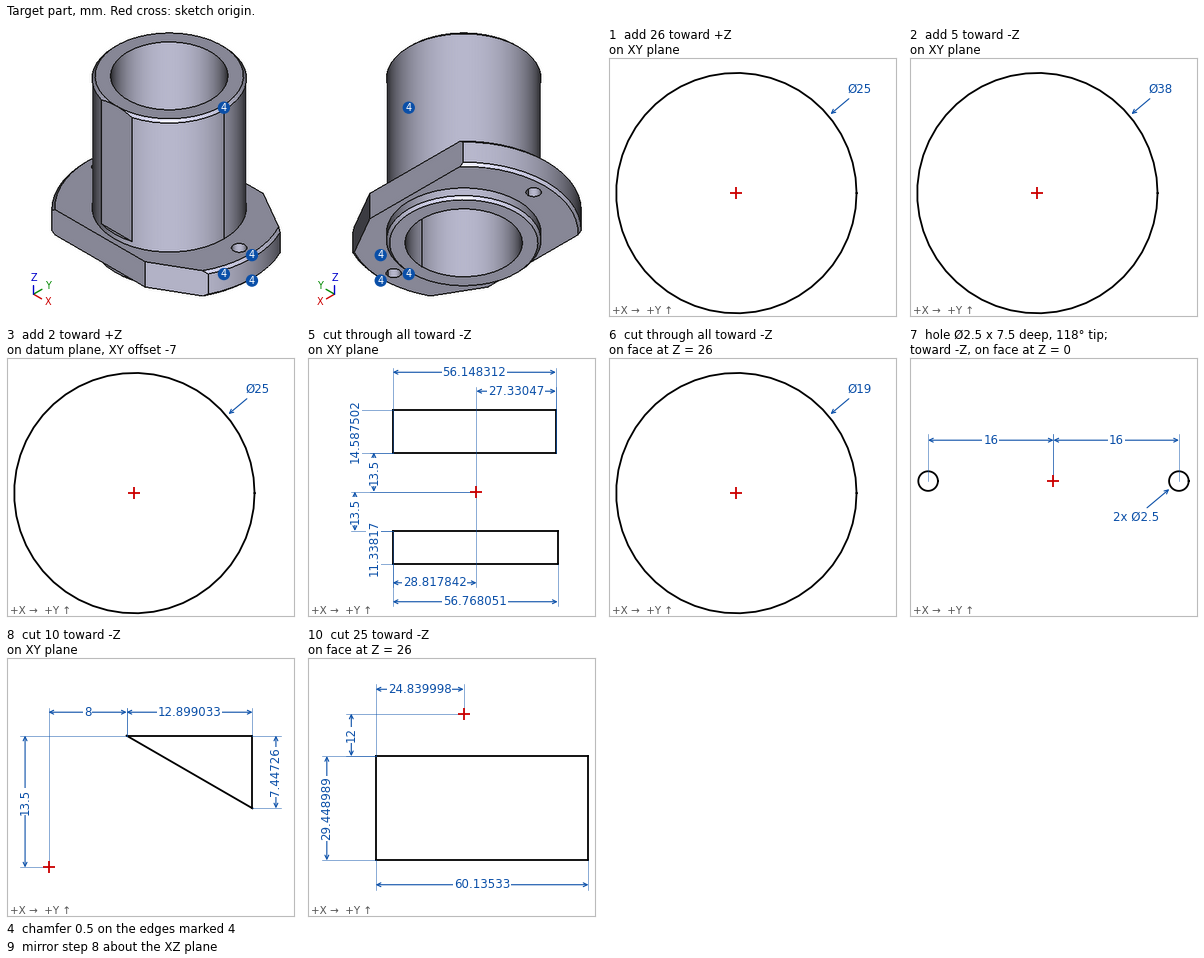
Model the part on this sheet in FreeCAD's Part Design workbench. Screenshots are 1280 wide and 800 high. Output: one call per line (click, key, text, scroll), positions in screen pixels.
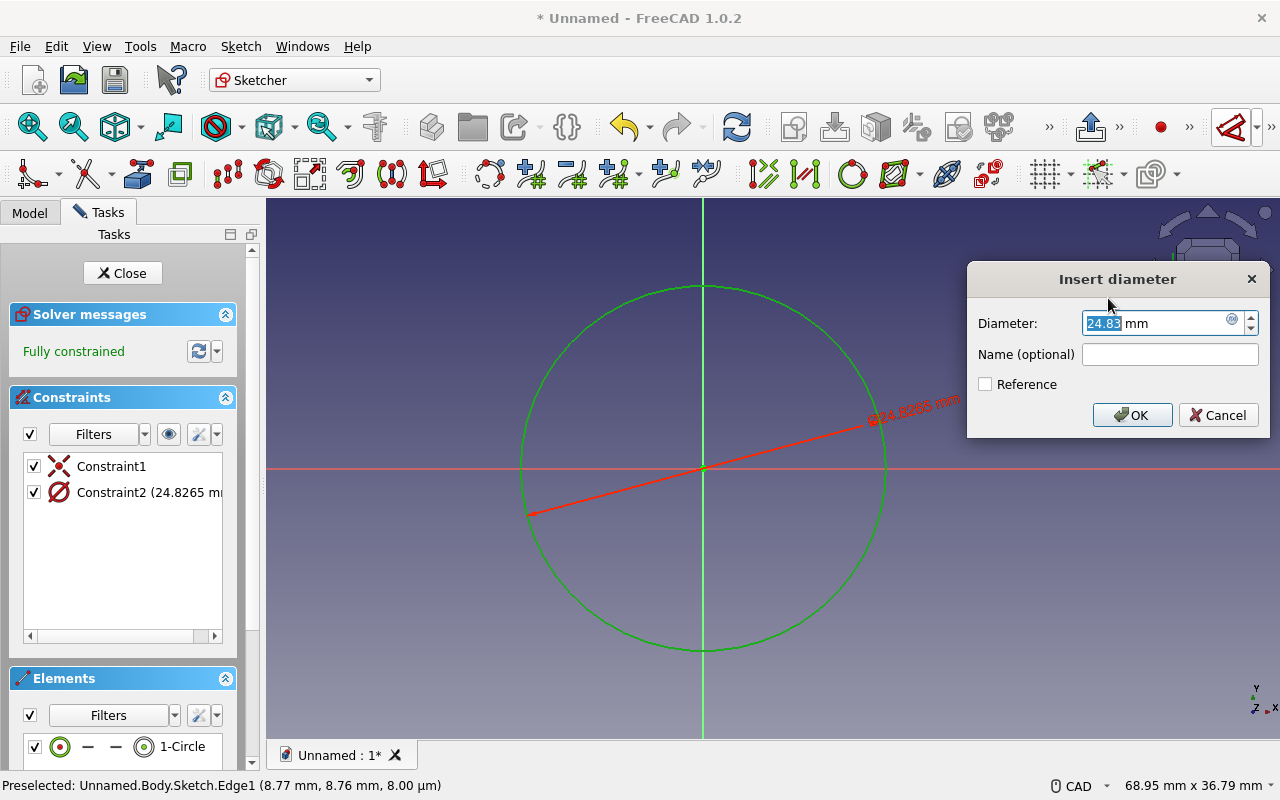
text(25)
key(Return)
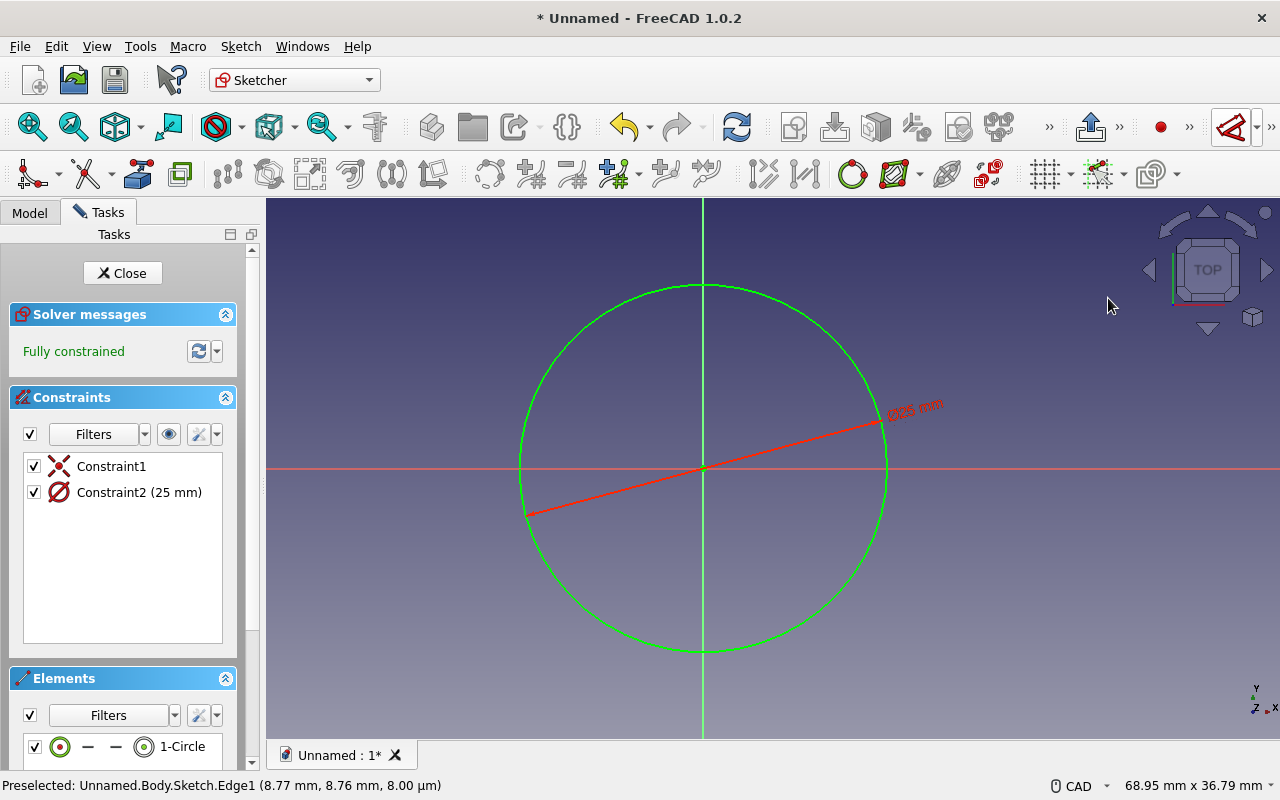
click(123, 273)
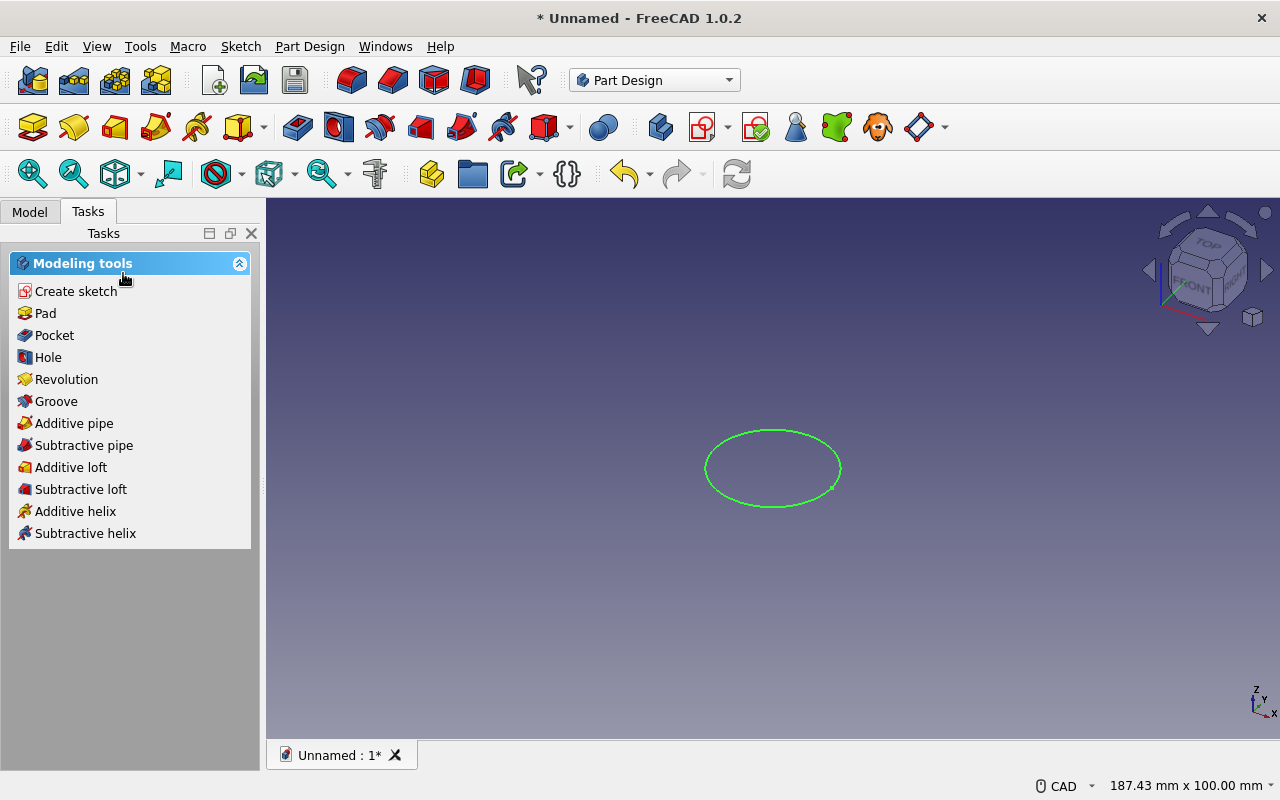
click(33, 128)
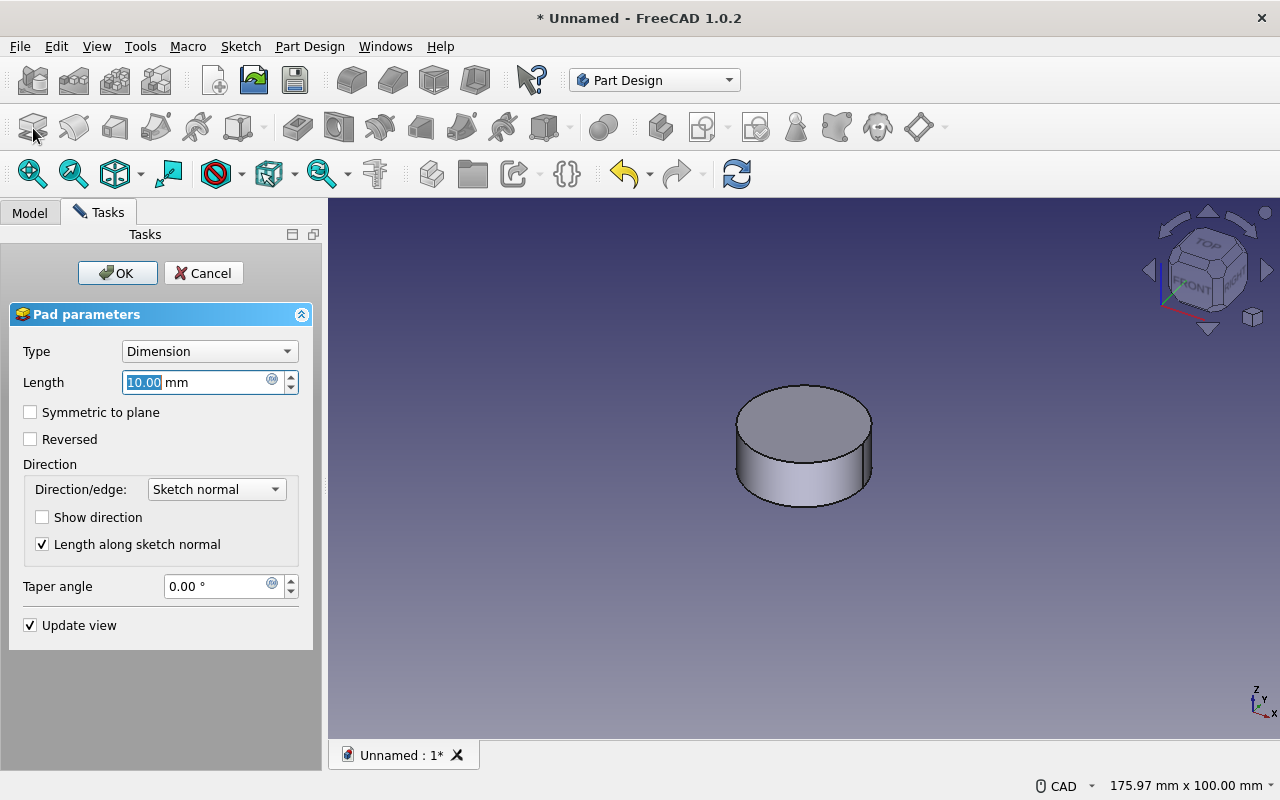
text(26)
key(Tab)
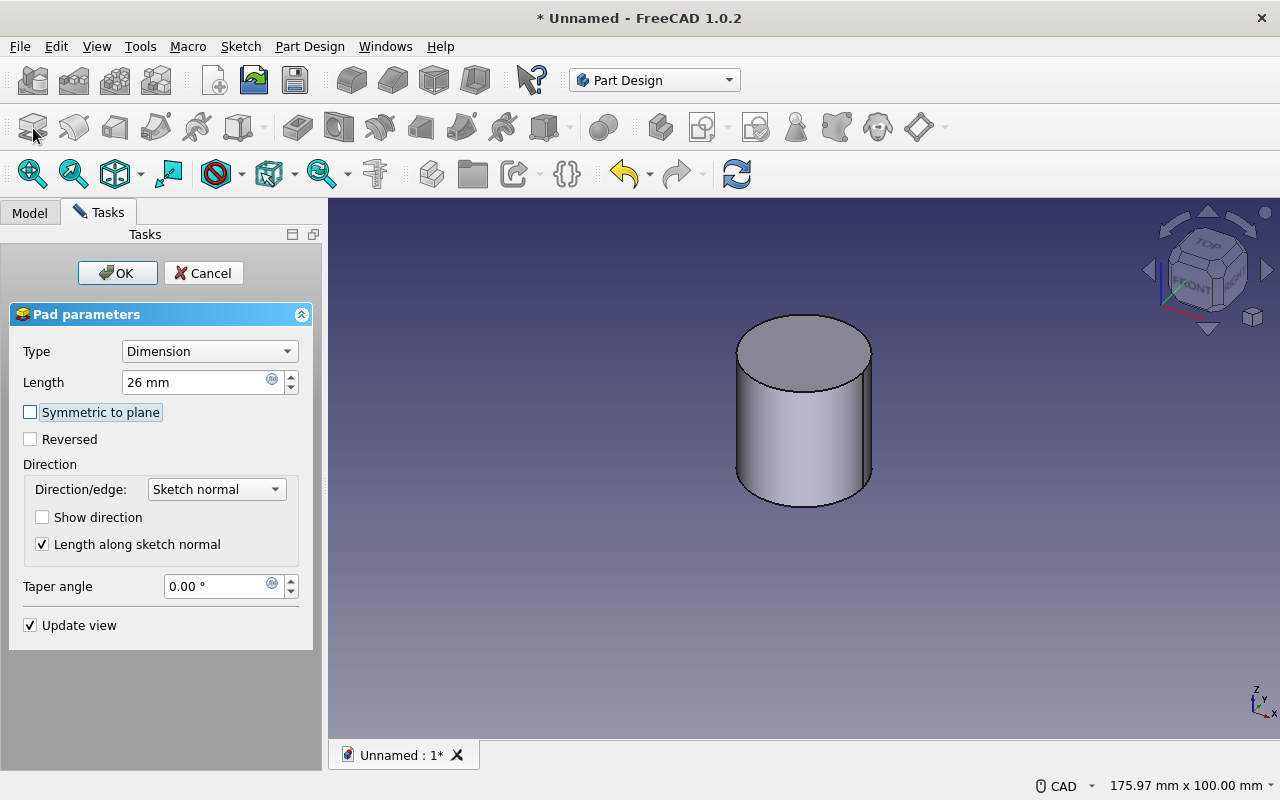
click(118, 273)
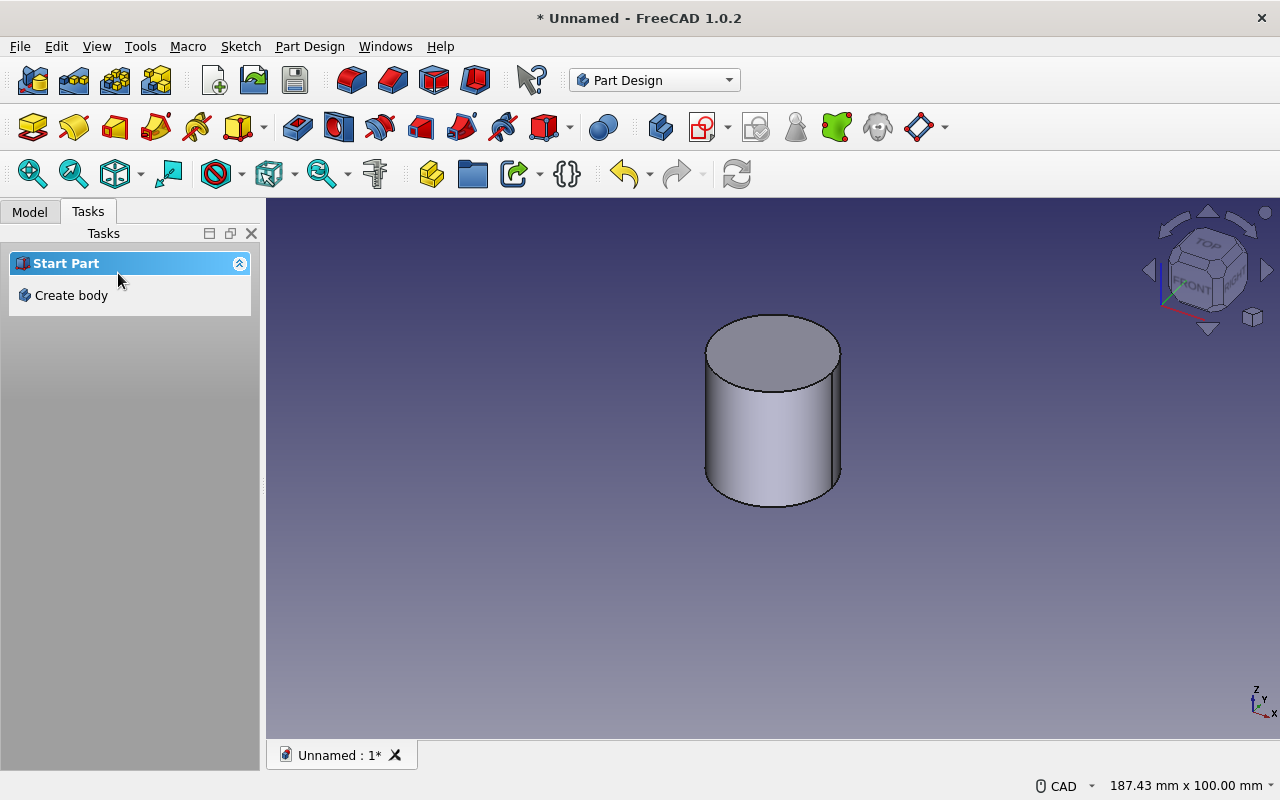
click(33, 174)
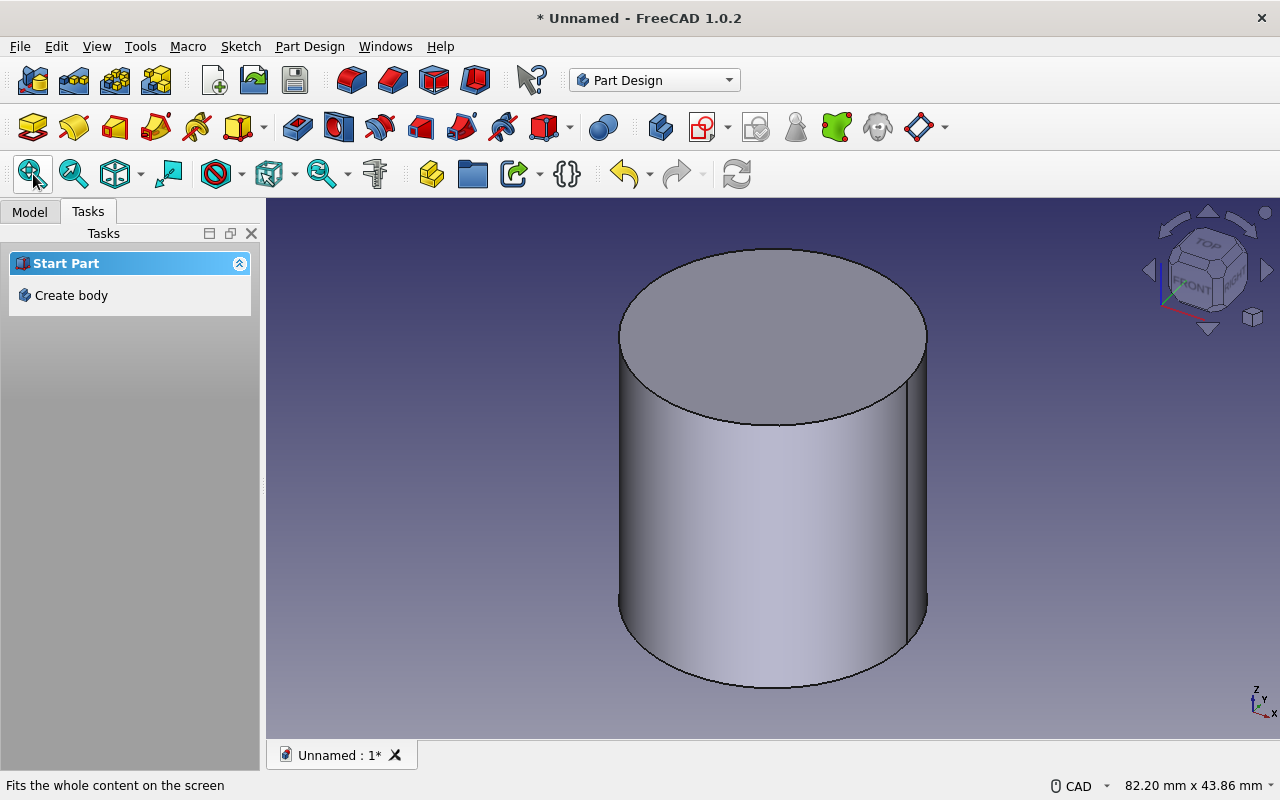
click(702, 128)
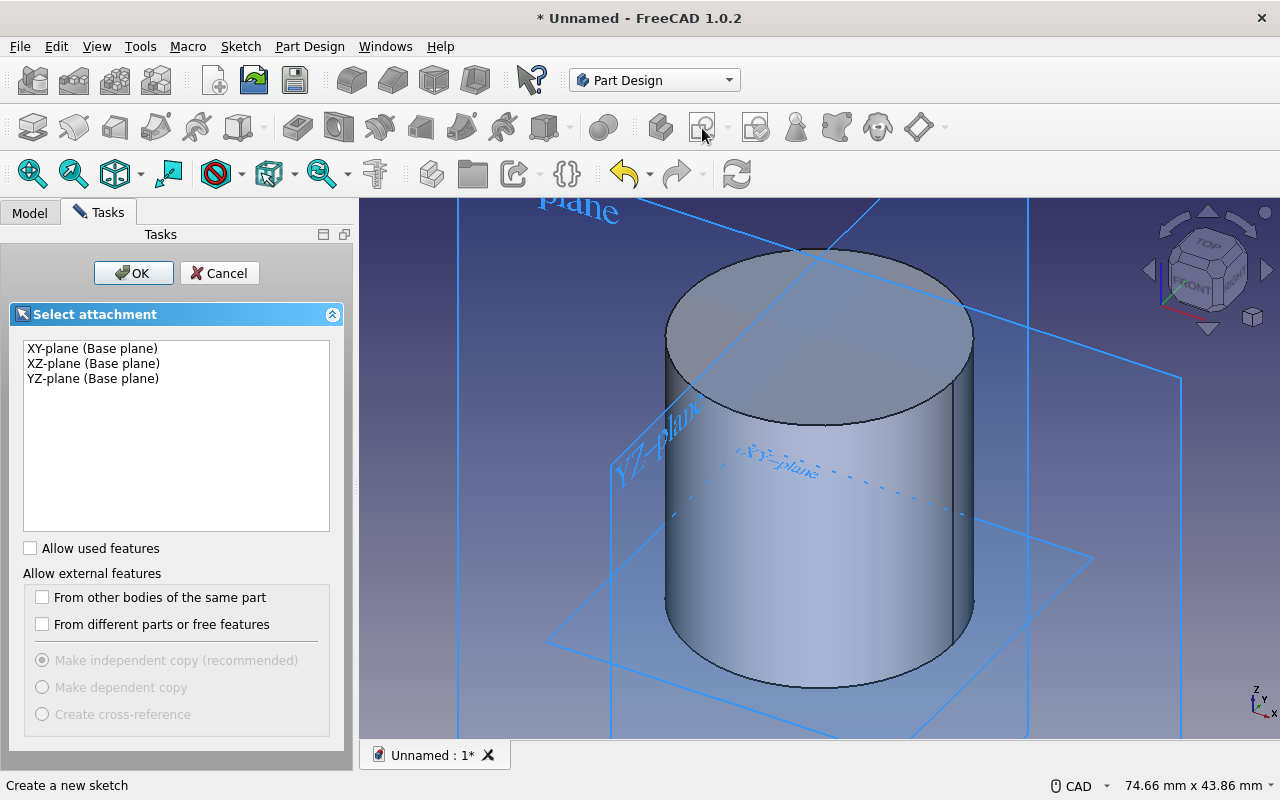
click(84, 348)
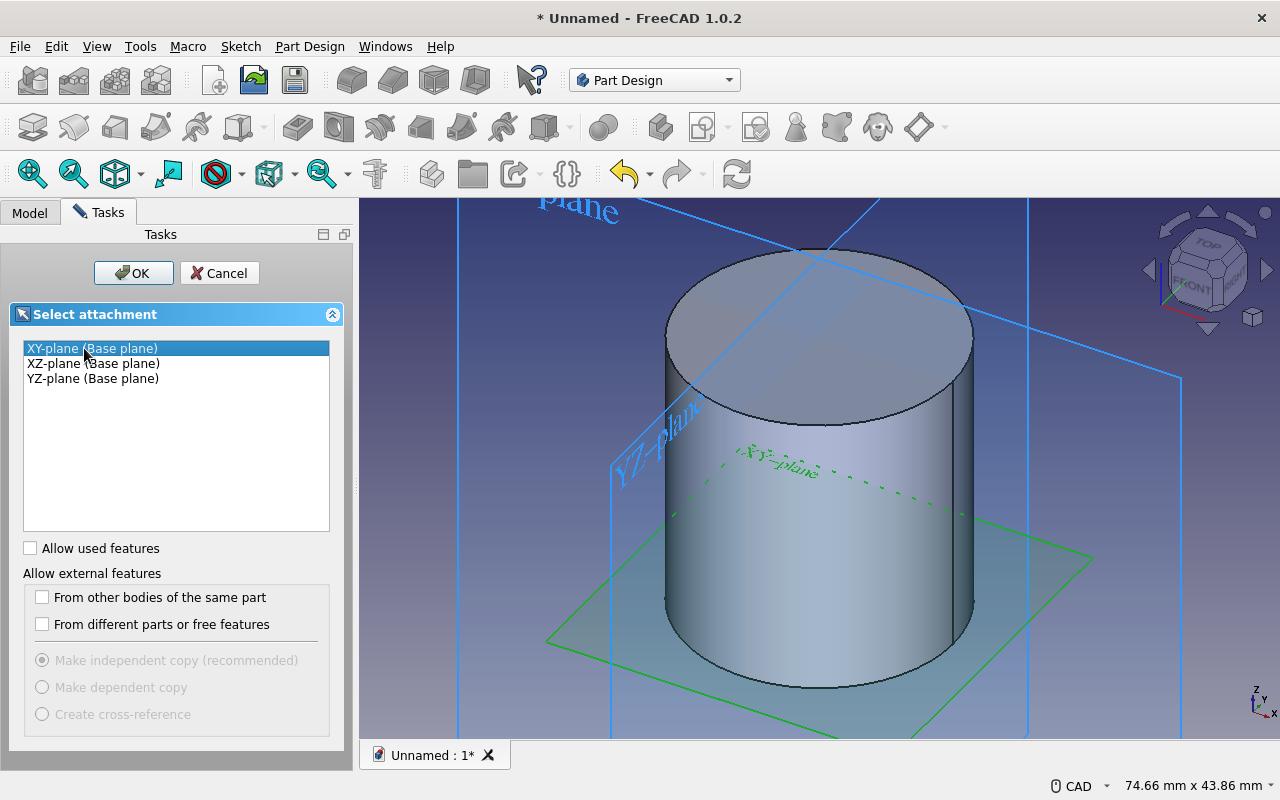
click(134, 273)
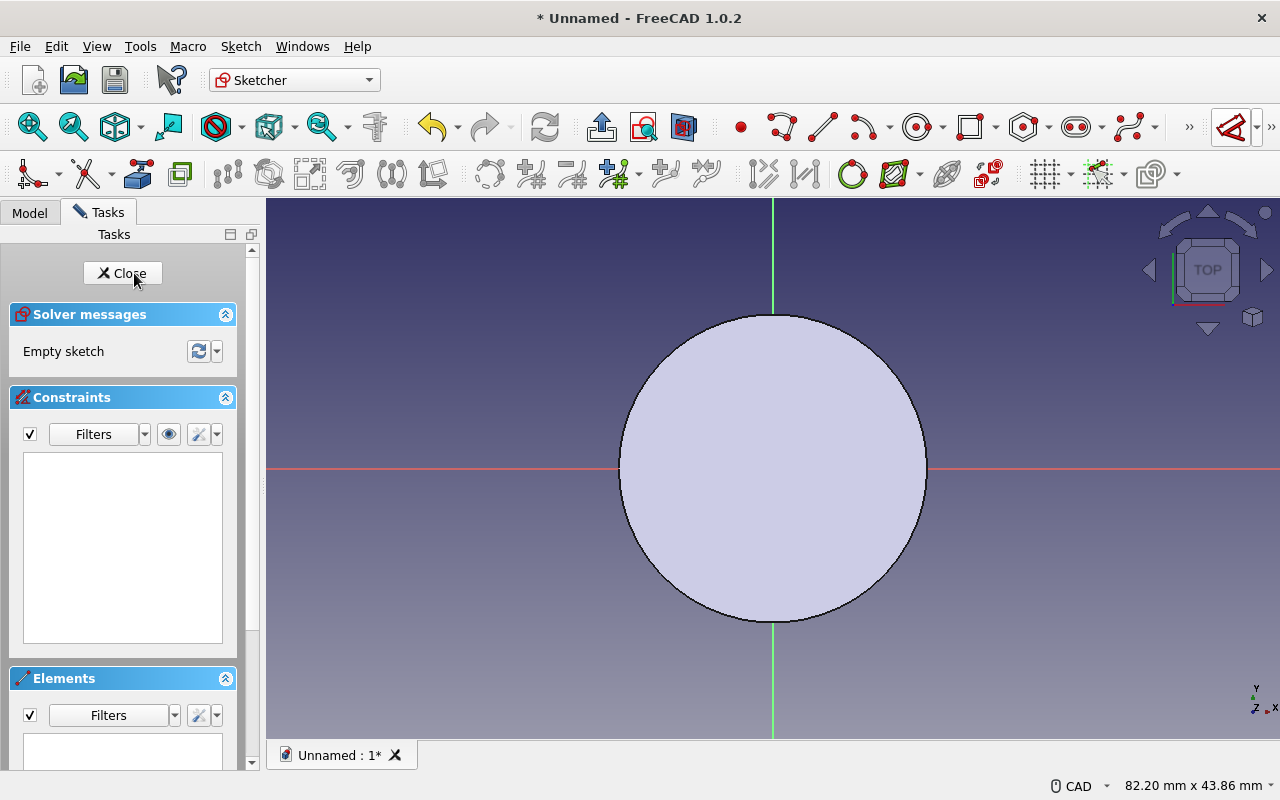
click(684, 128)